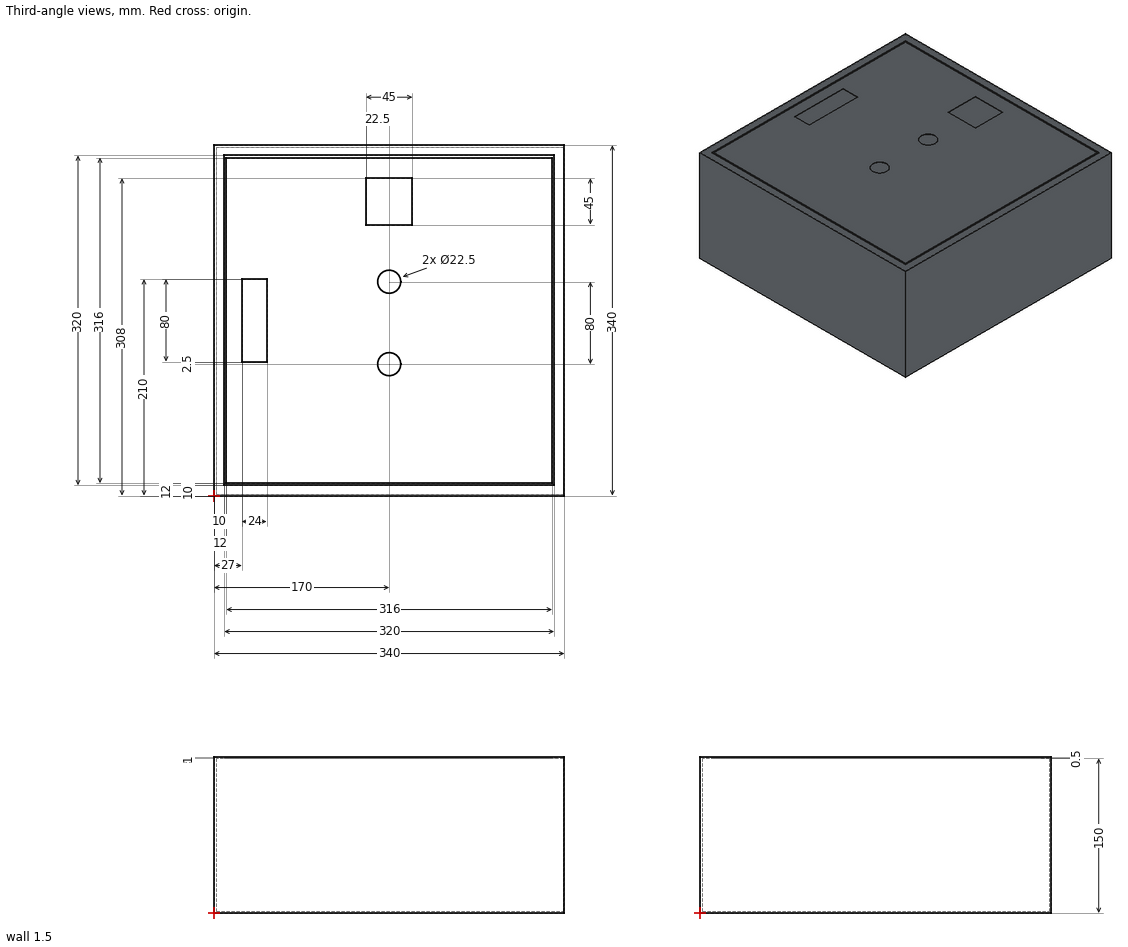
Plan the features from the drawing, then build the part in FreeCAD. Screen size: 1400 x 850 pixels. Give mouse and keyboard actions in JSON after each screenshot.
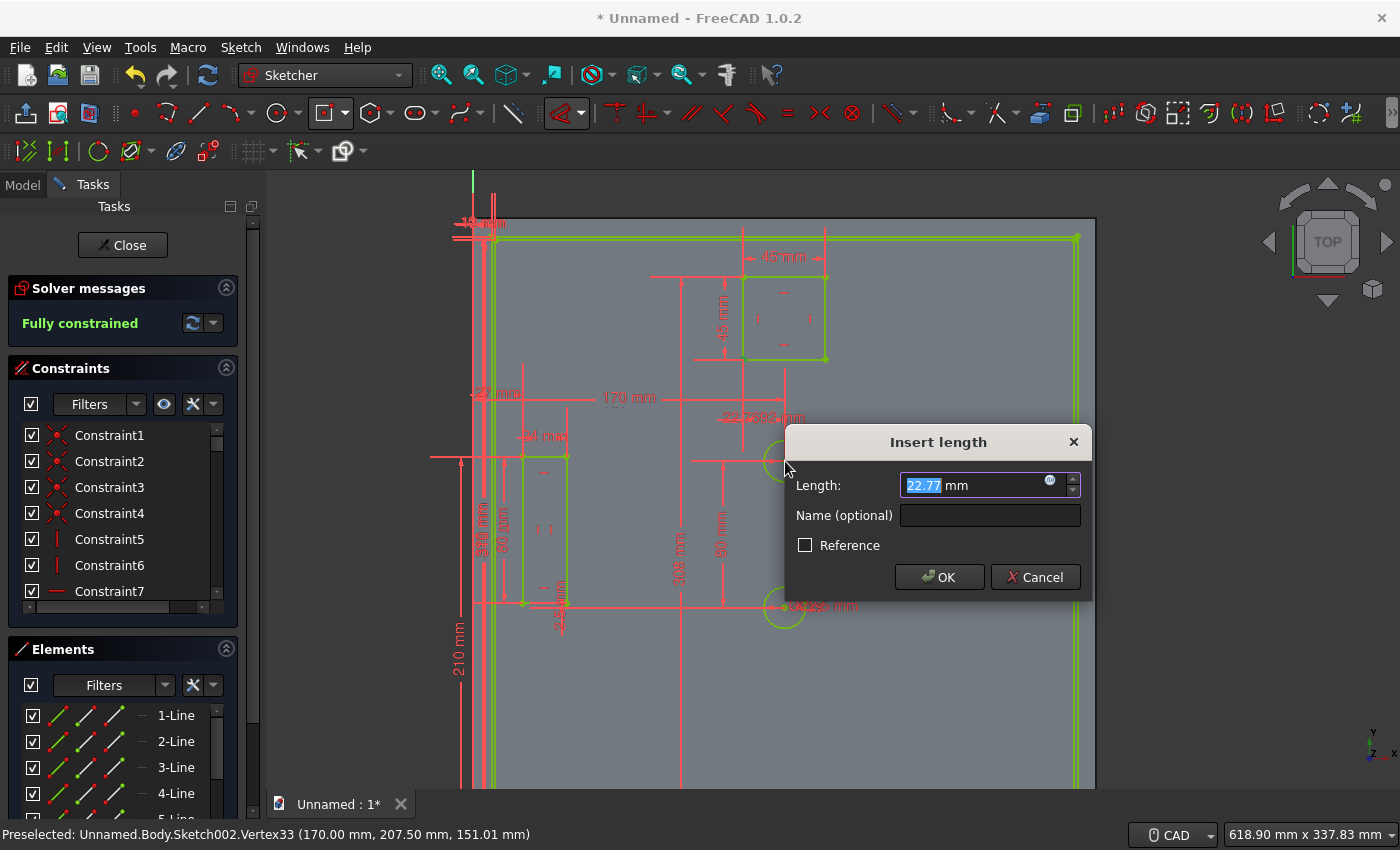
{"action": "type", "text": "22.5"}
{"action": "key", "text": "Return"}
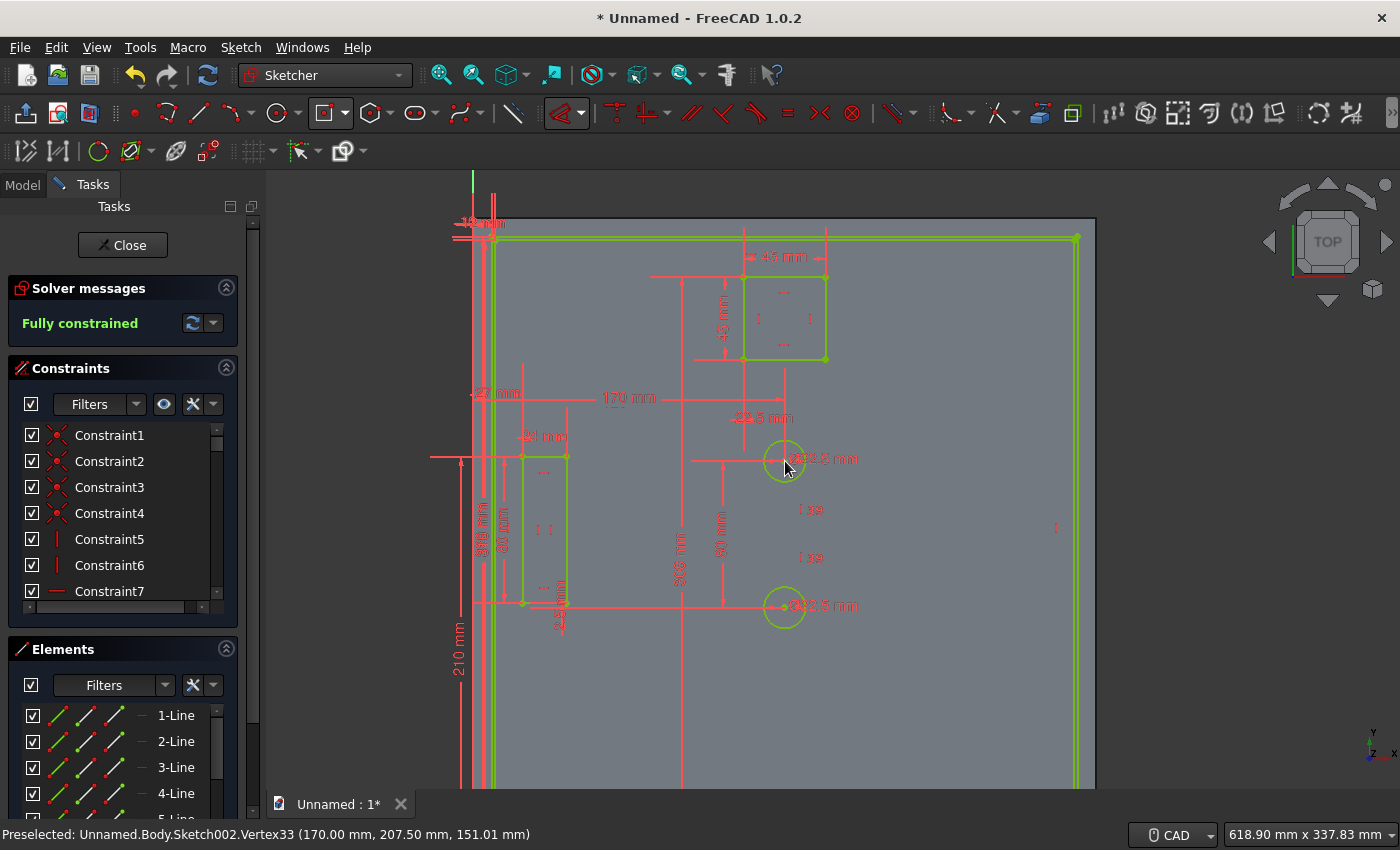
{"action": "left_click", "coordinate": [123, 245]}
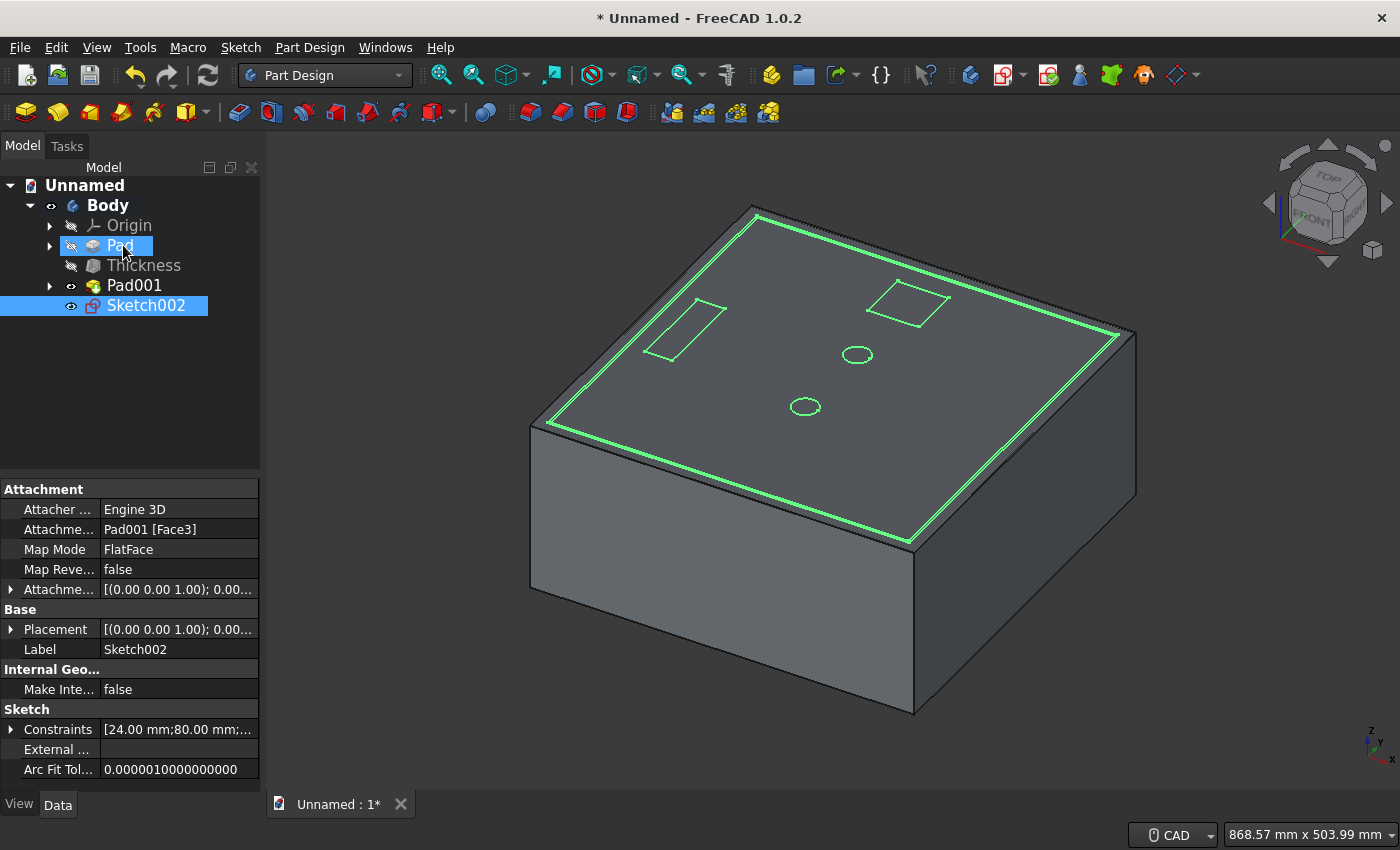
{"action": "left_click", "coordinate": [240, 112]}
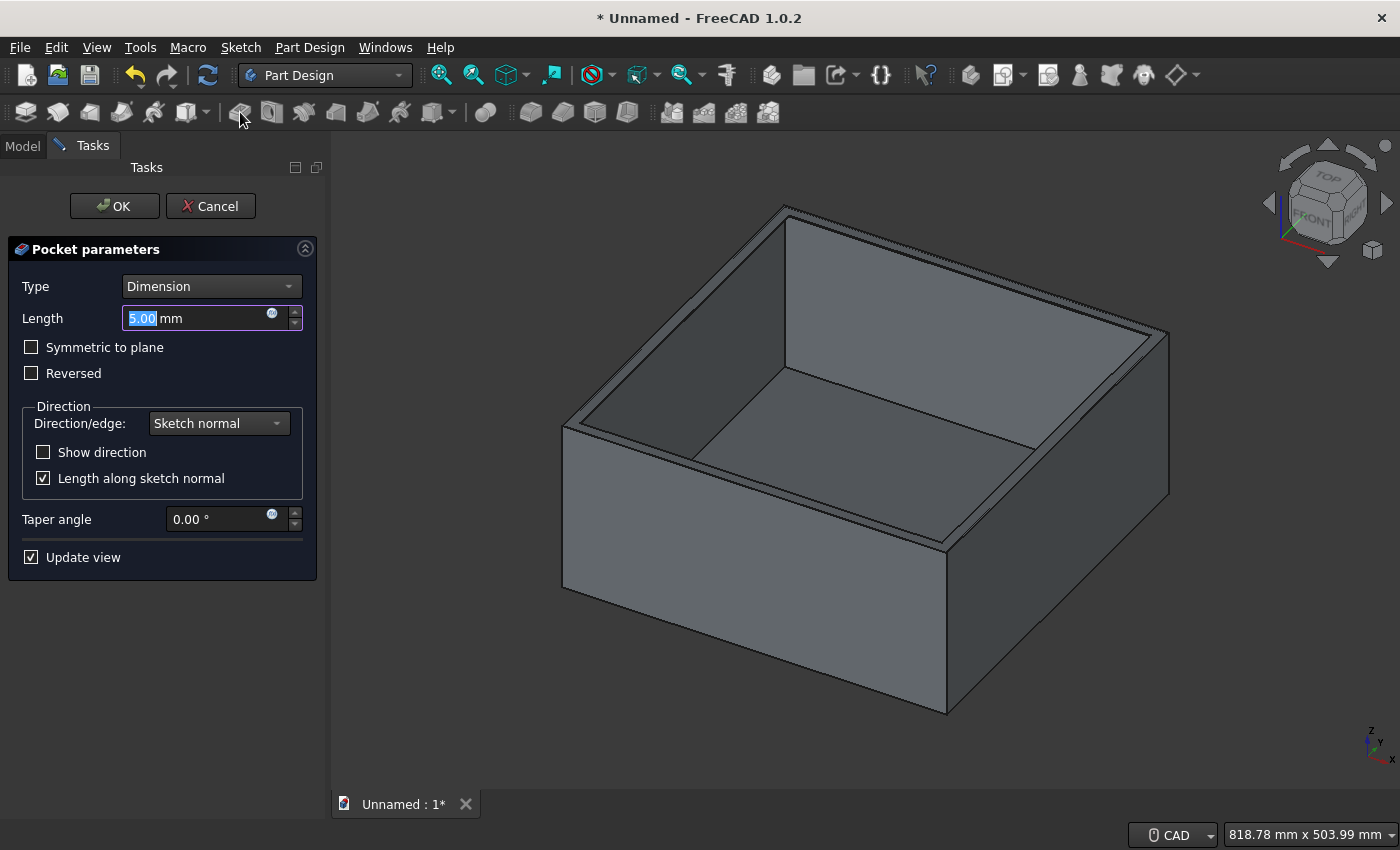
{"action": "type", "text": "0.5"}
{"action": "key", "text": "Tab"}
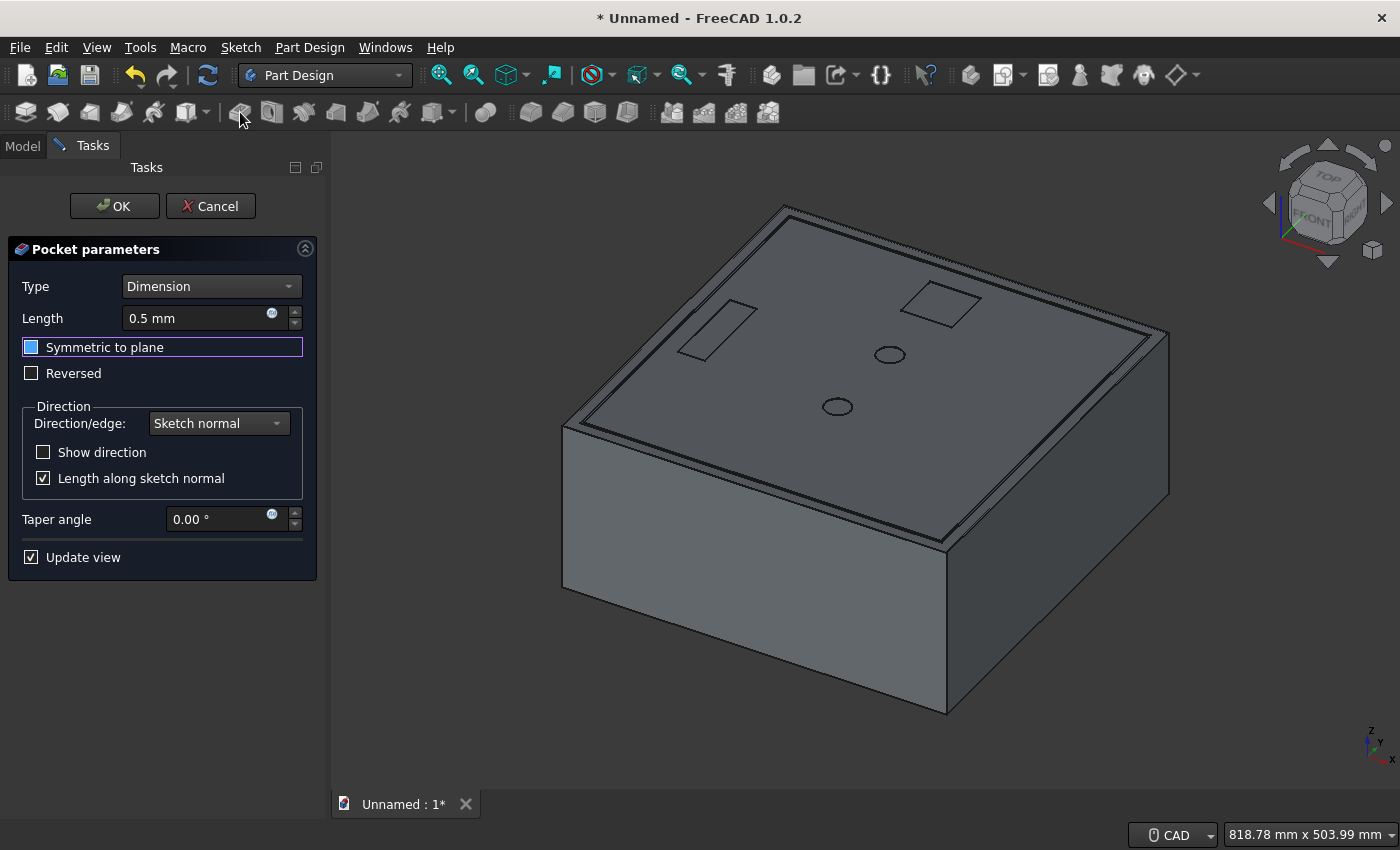
{"action": "left_click", "coordinate": [115, 206]}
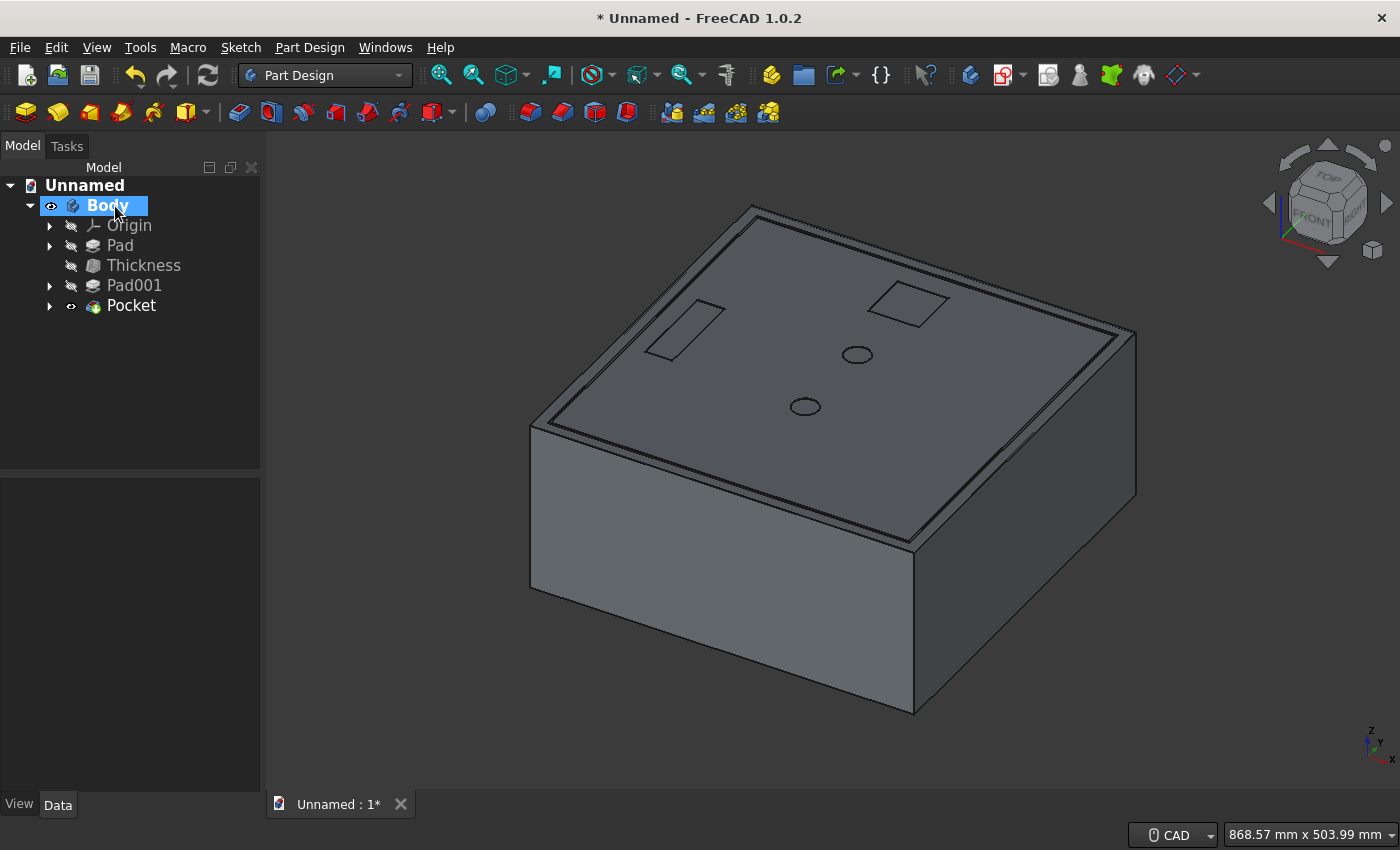
{"action": "key", "text": "0"}